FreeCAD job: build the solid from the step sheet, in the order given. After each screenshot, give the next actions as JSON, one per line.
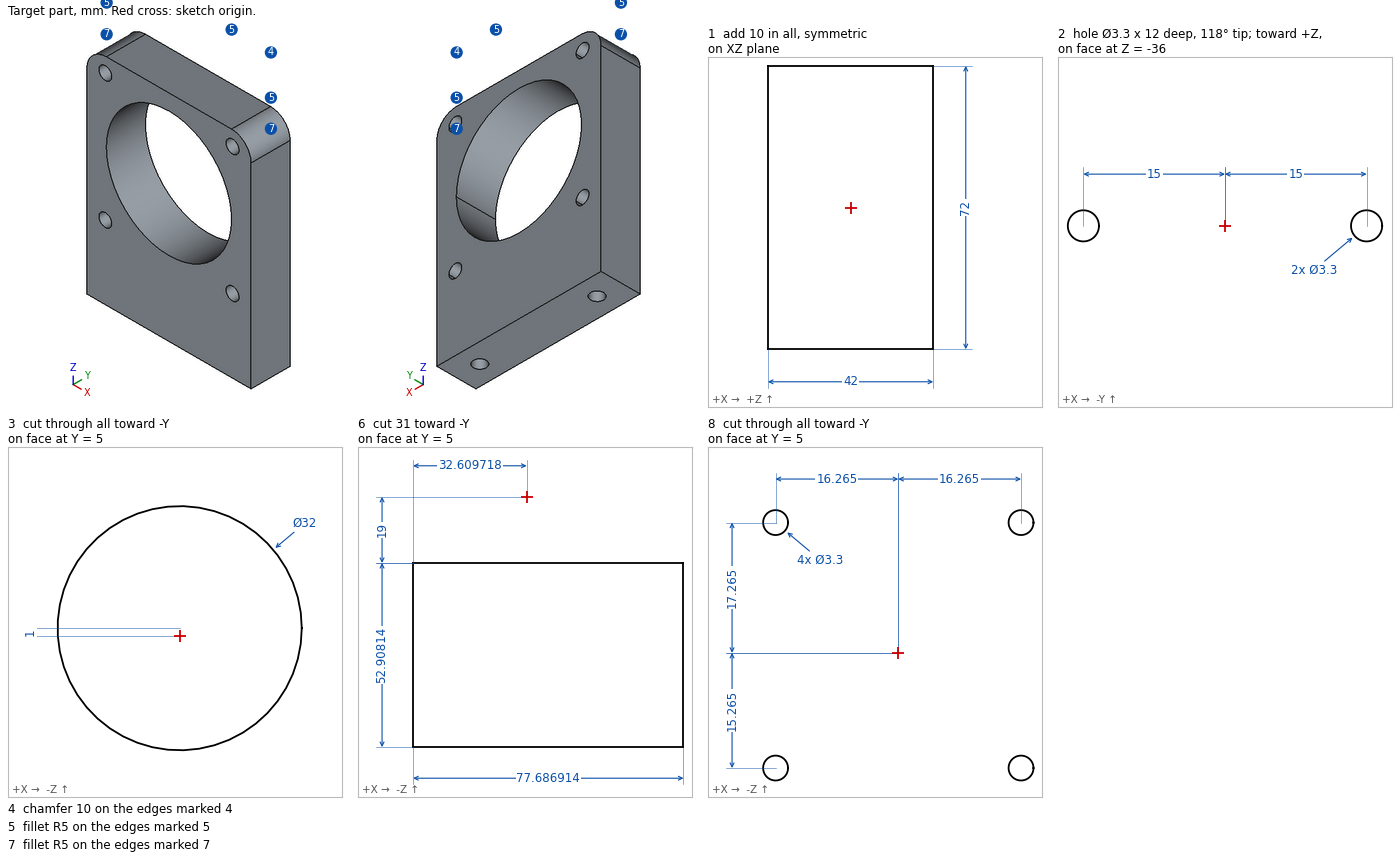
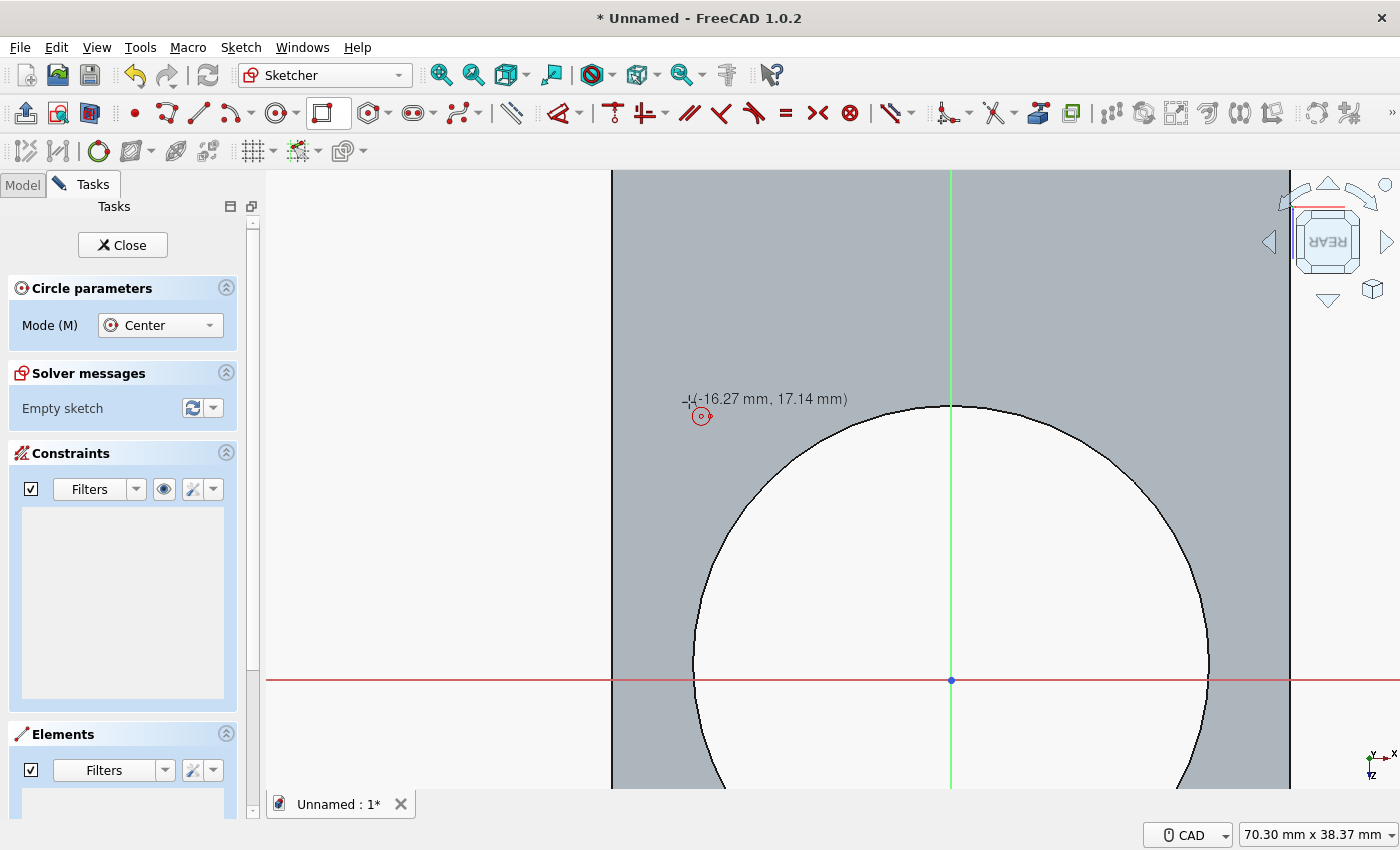
{"action": "left_click", "coordinate": [689, 402]}
{"action": "left_click", "coordinate": [708, 383]}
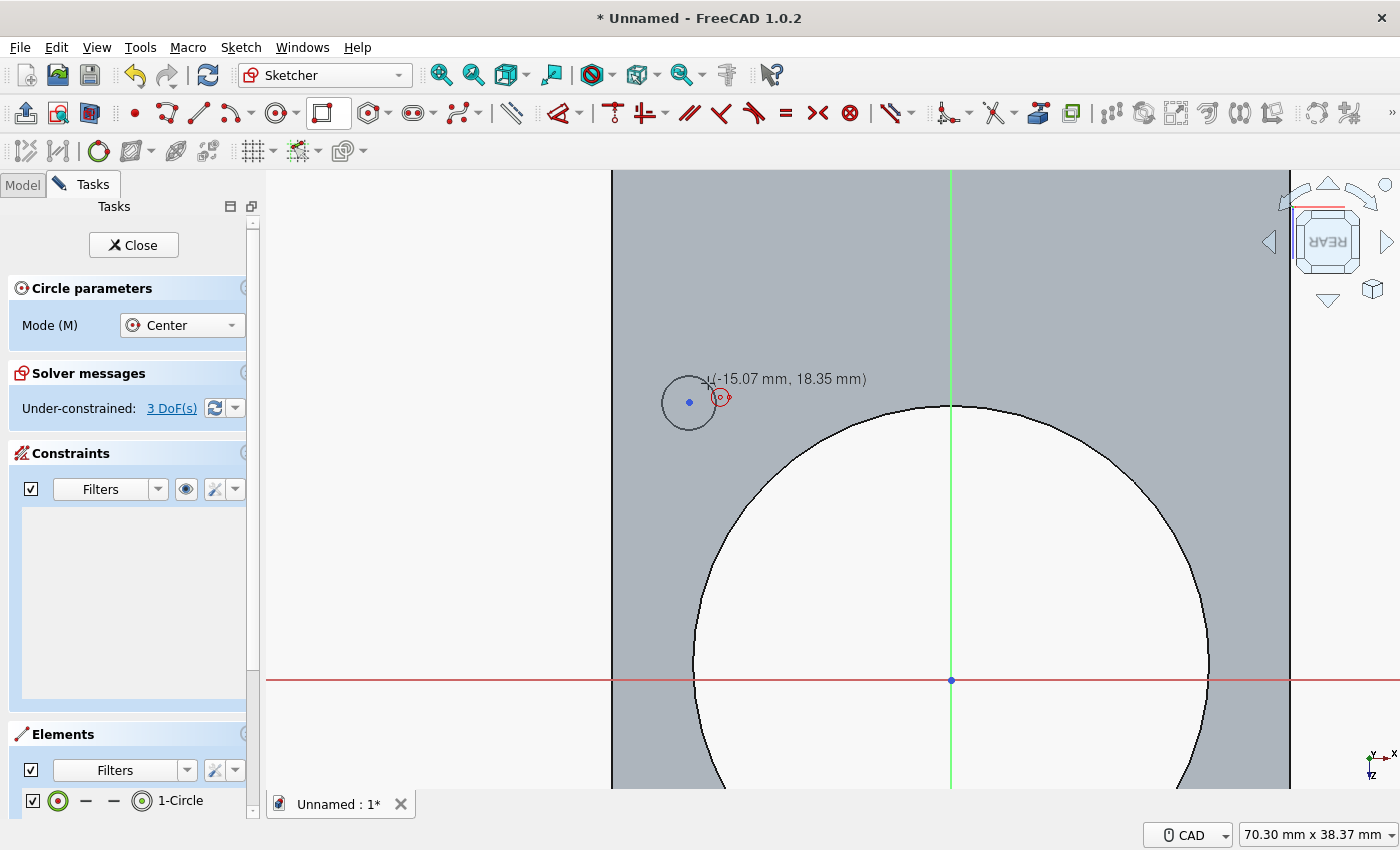
{"action": "left_click", "coordinate": [1213, 402]}
{"action": "left_click", "coordinate": [1232, 383]}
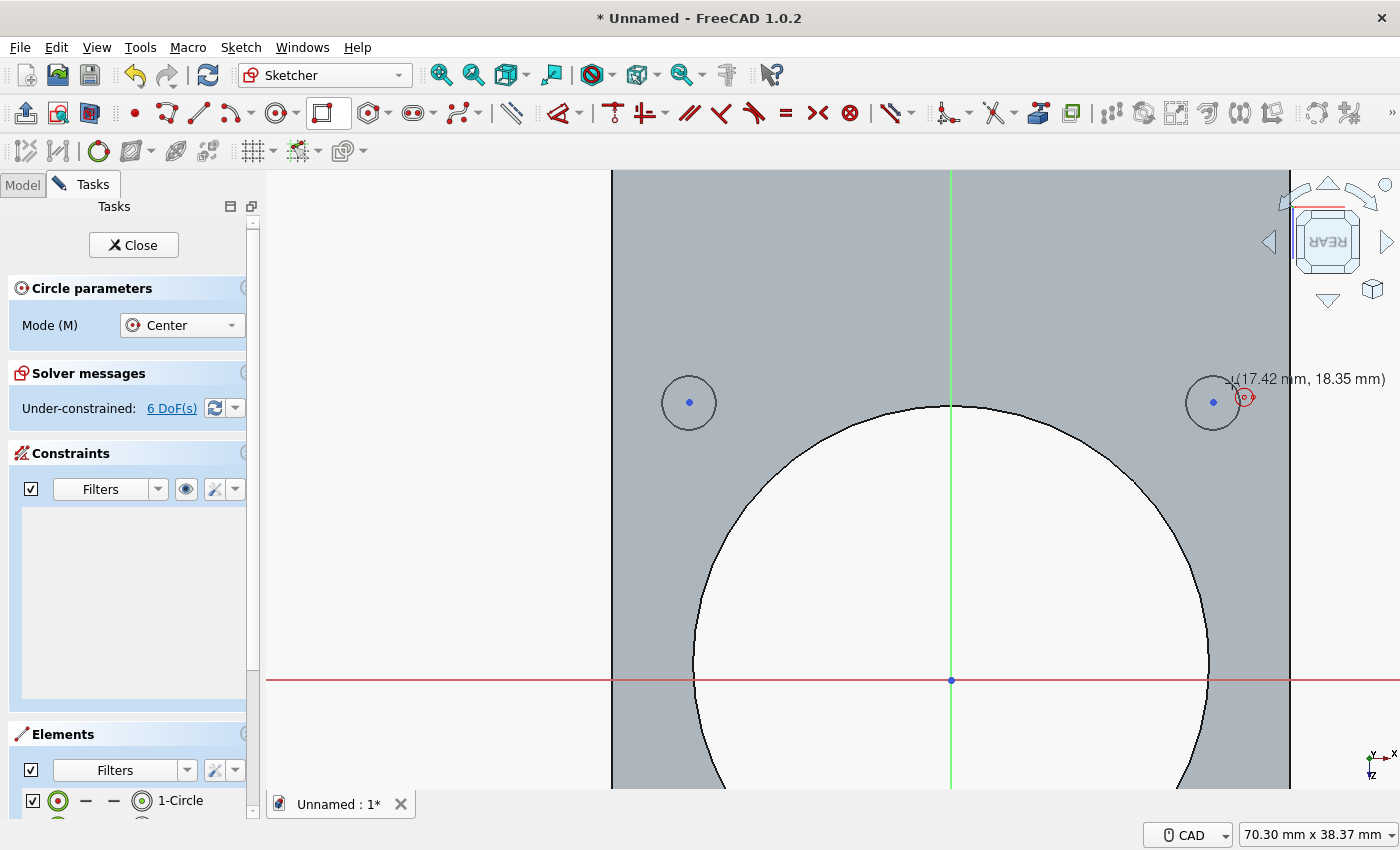
{"action": "scroll", "coordinate": [385, 198], "scroll_direction": "down", "scroll_amount": 2}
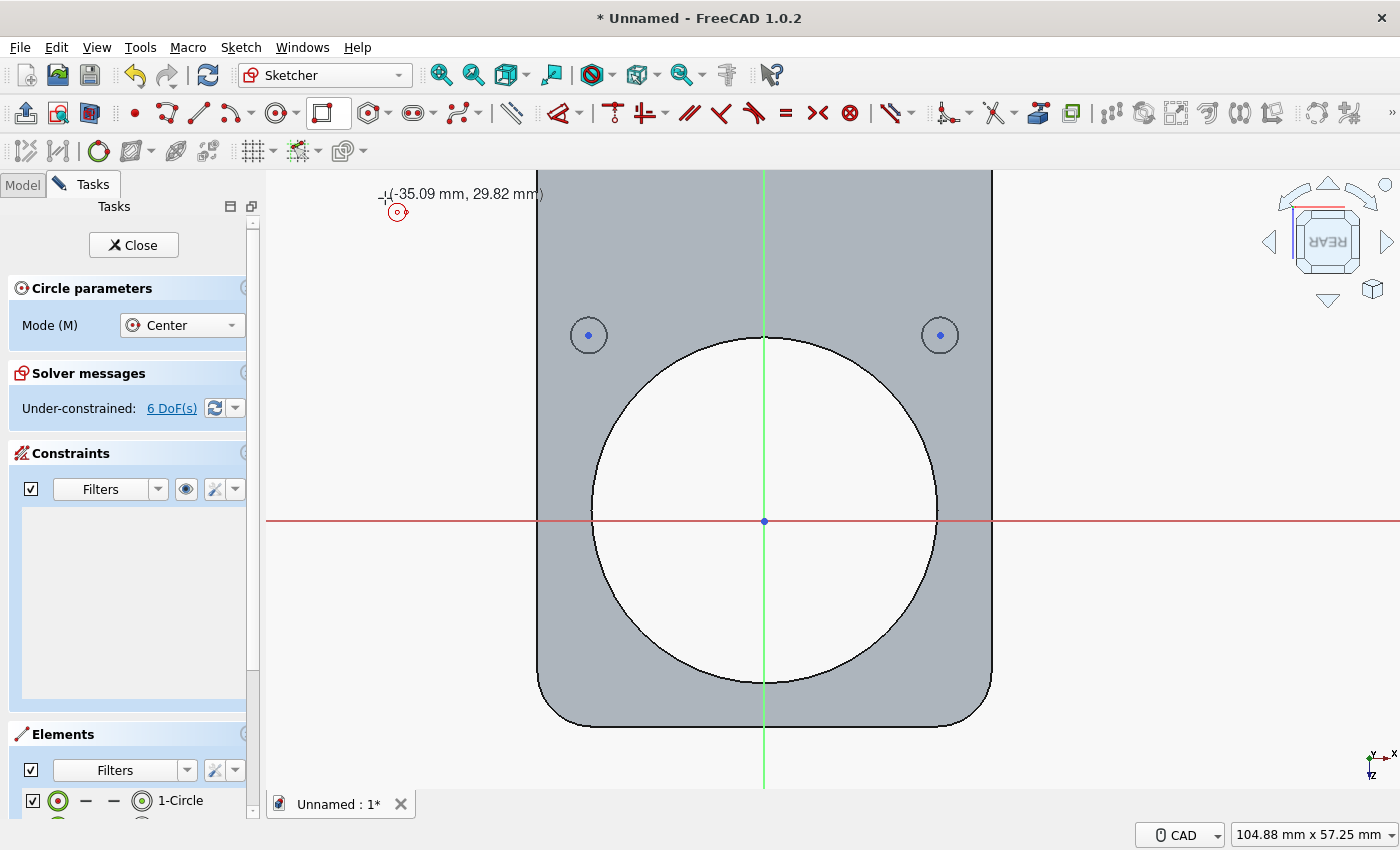
{"action": "scroll", "coordinate": [589, 686], "scroll_direction": "up", "scroll_amount": 2}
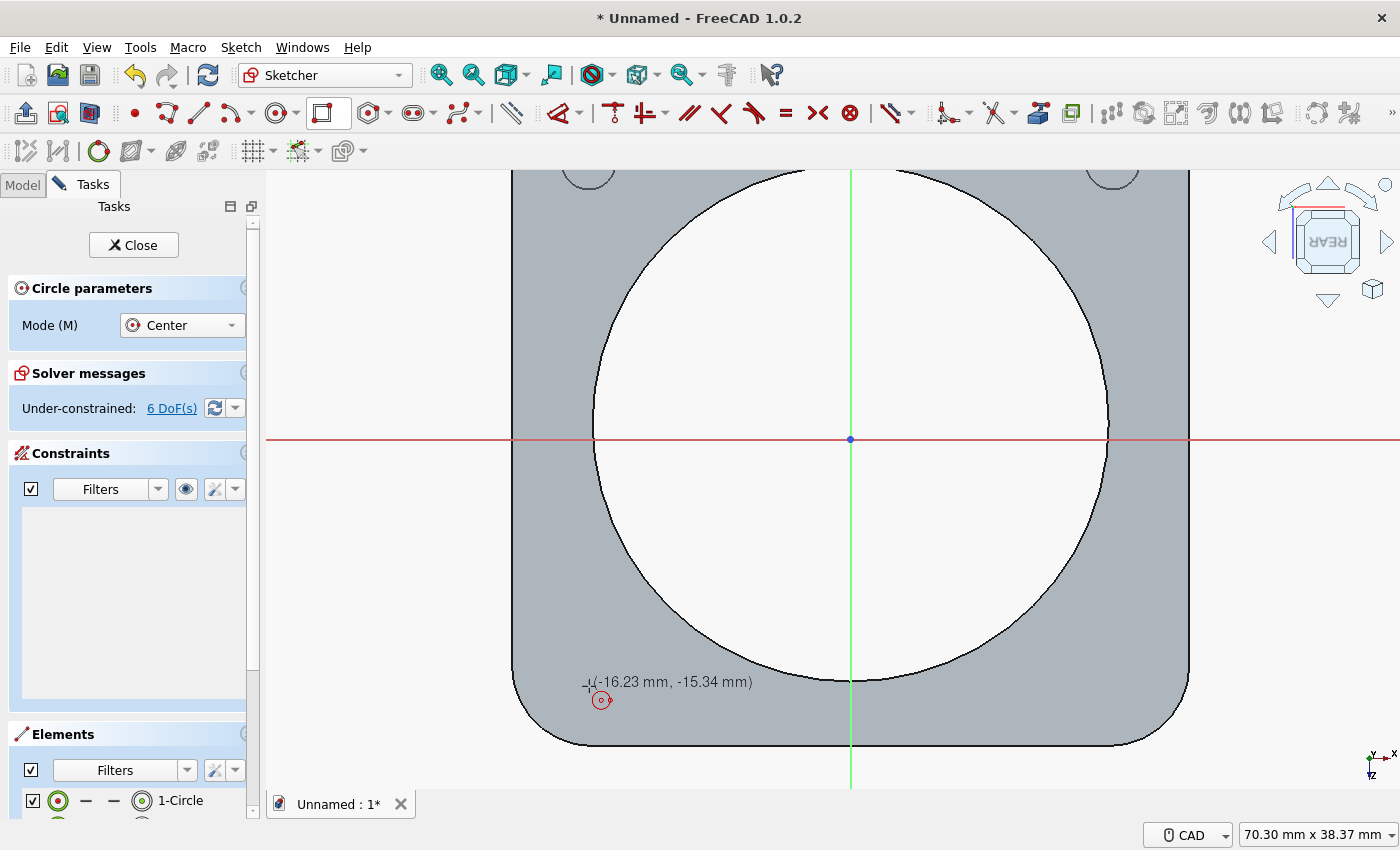
{"action": "left_click", "coordinate": [588, 686]}
{"action": "left_click", "coordinate": [607, 667]}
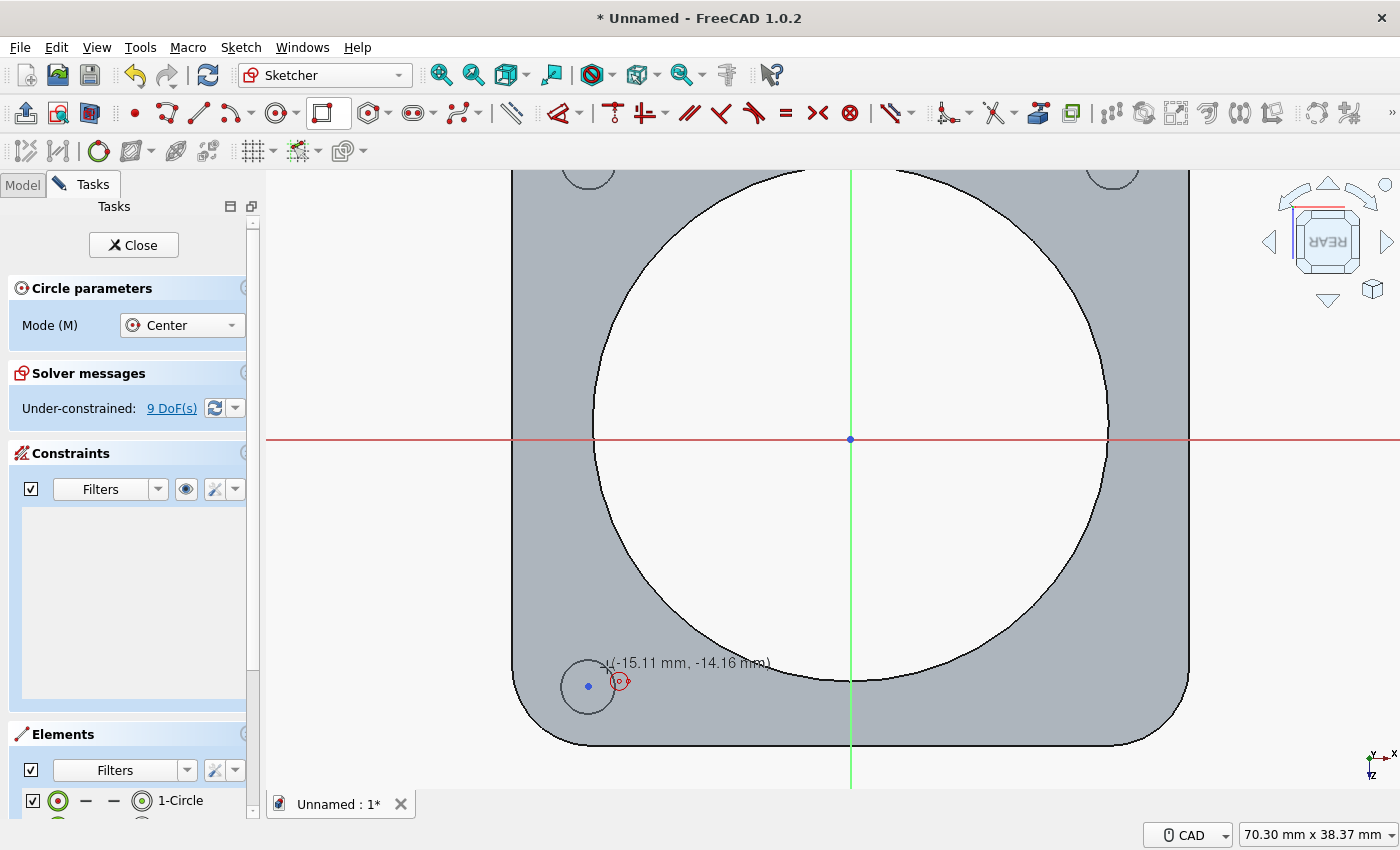
{"action": "left_click", "coordinate": [1113, 686]}
{"action": "left_click", "coordinate": [1132, 667]}
{"action": "key", "text": "Escape"}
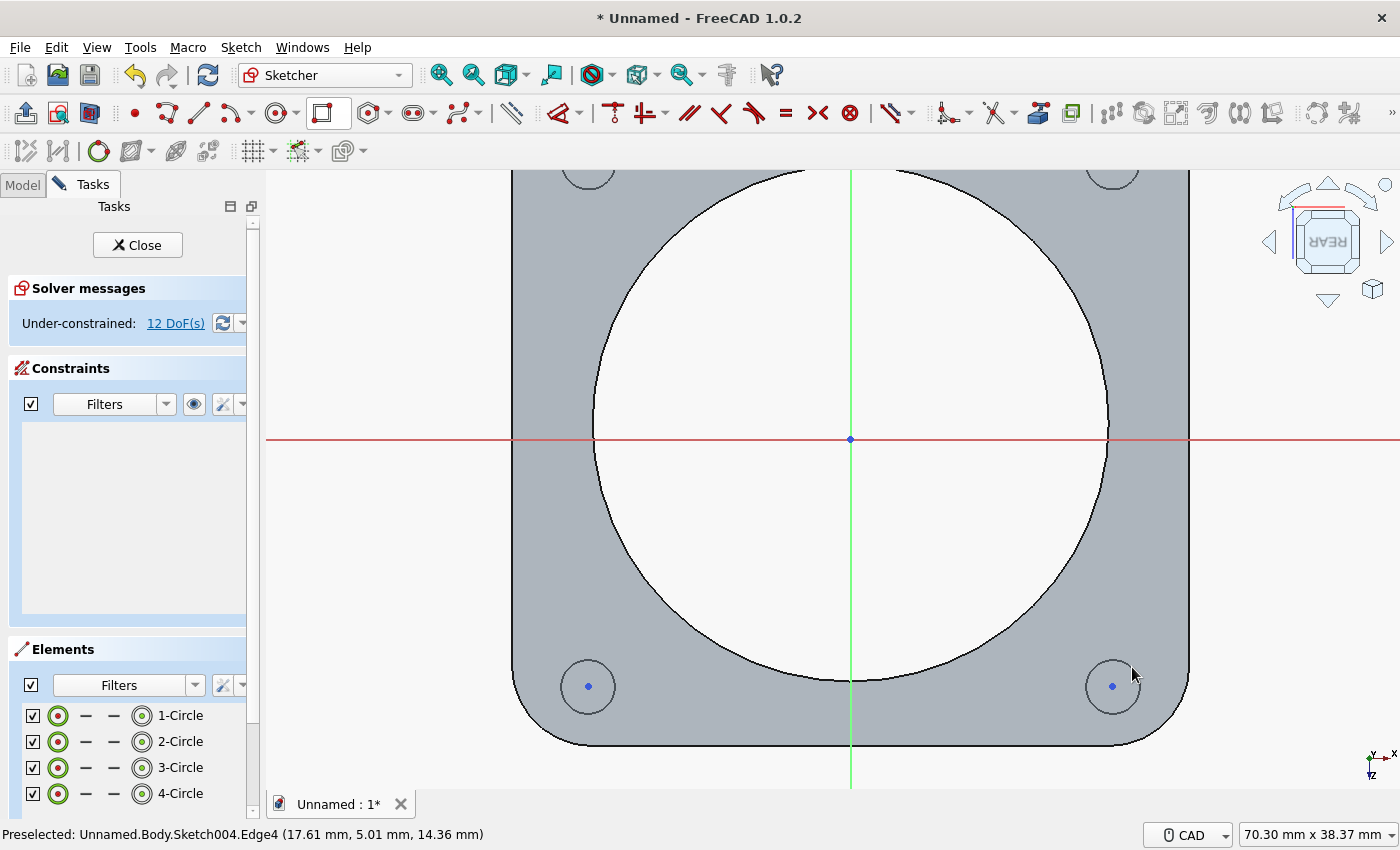
{"action": "scroll", "coordinate": [589, 593], "scroll_direction": "down", "scroll_amount": 2}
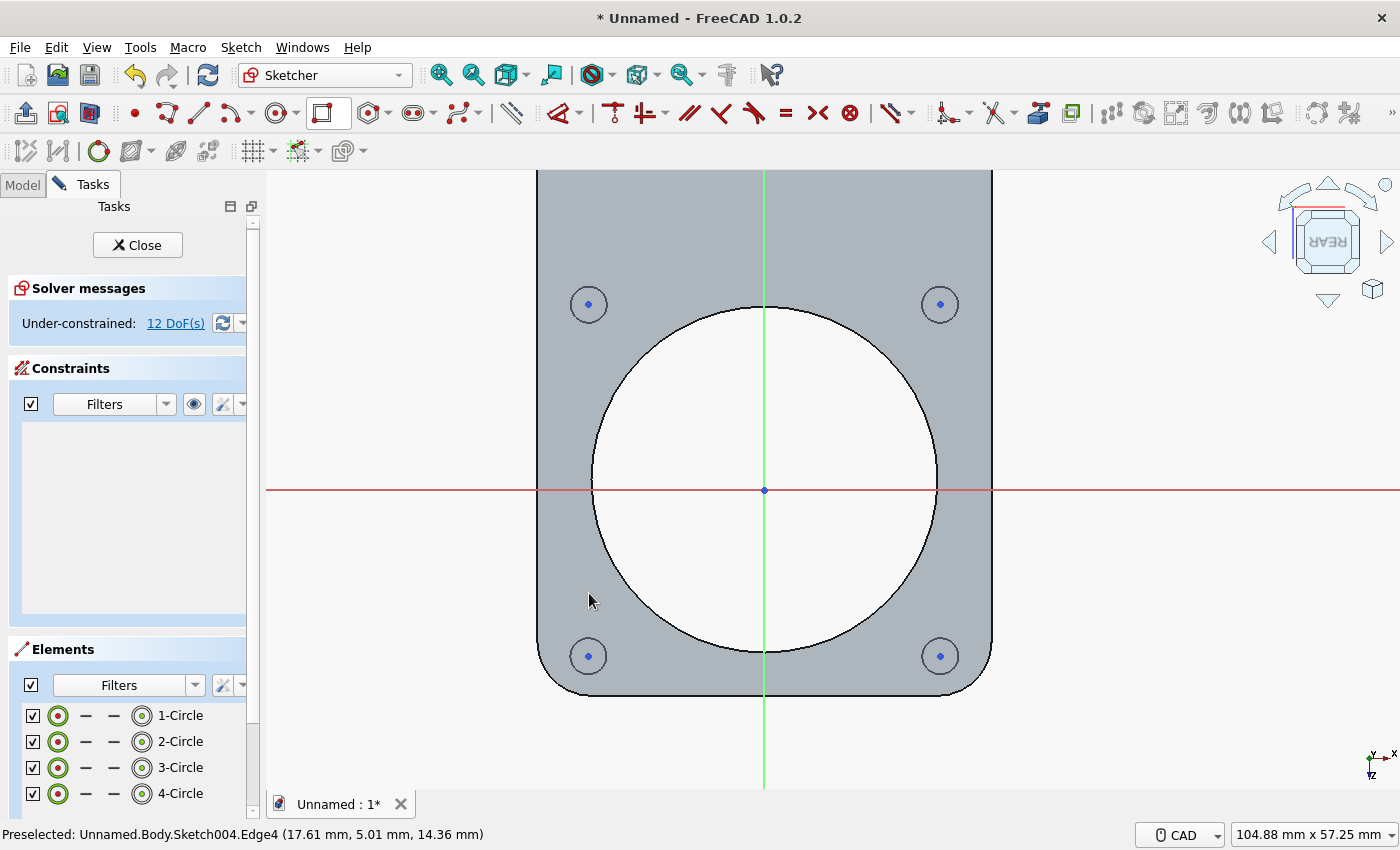
{"action": "left_click", "coordinate": [602, 292]}